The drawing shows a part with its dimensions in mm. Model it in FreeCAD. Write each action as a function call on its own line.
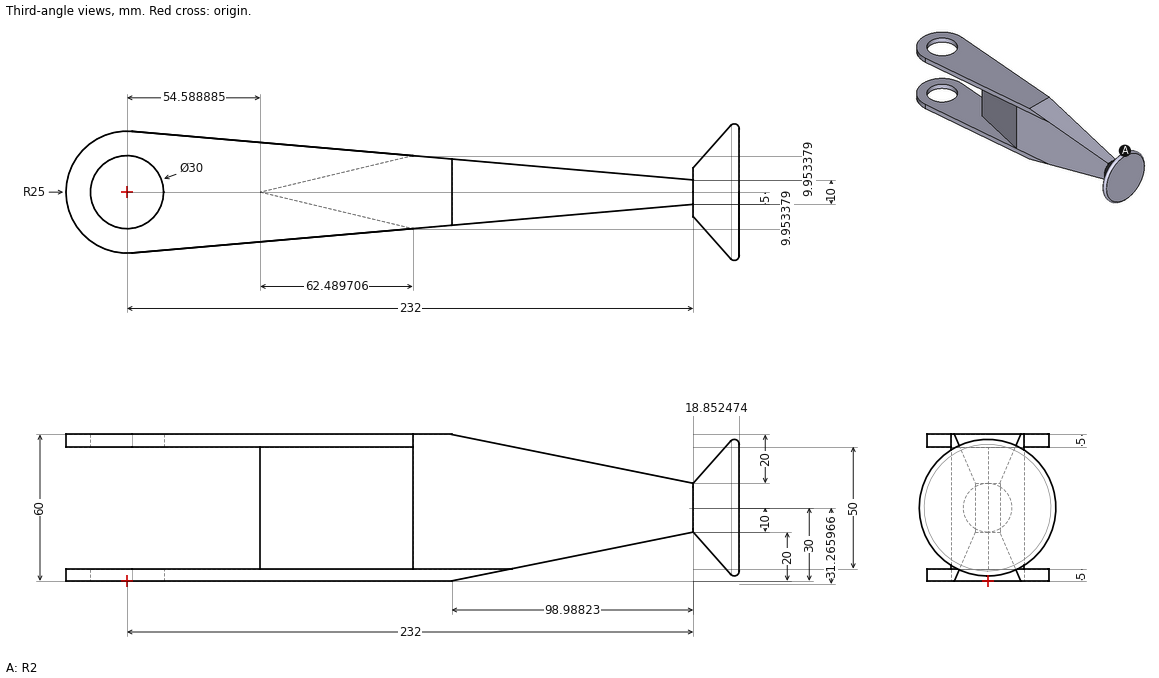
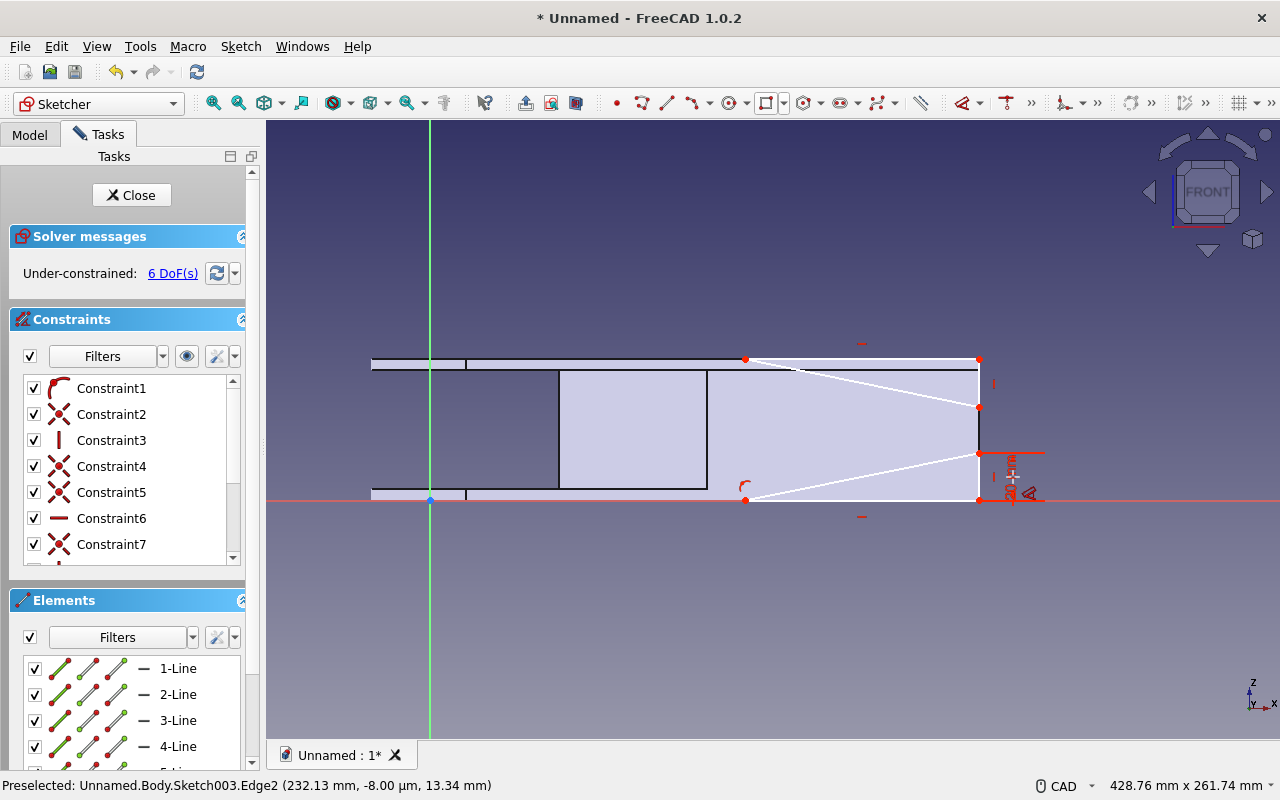
click(979, 374)
click(1013, 383)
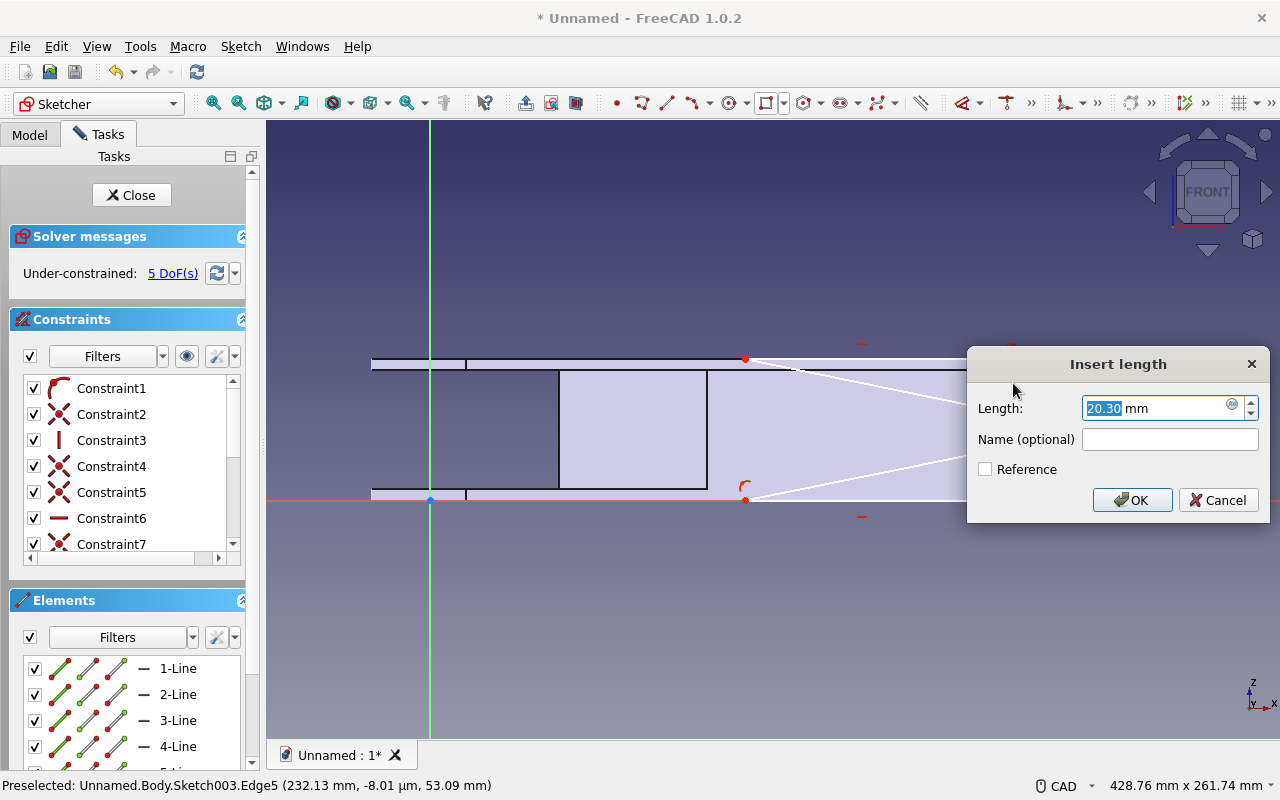
text(20)
key(Return)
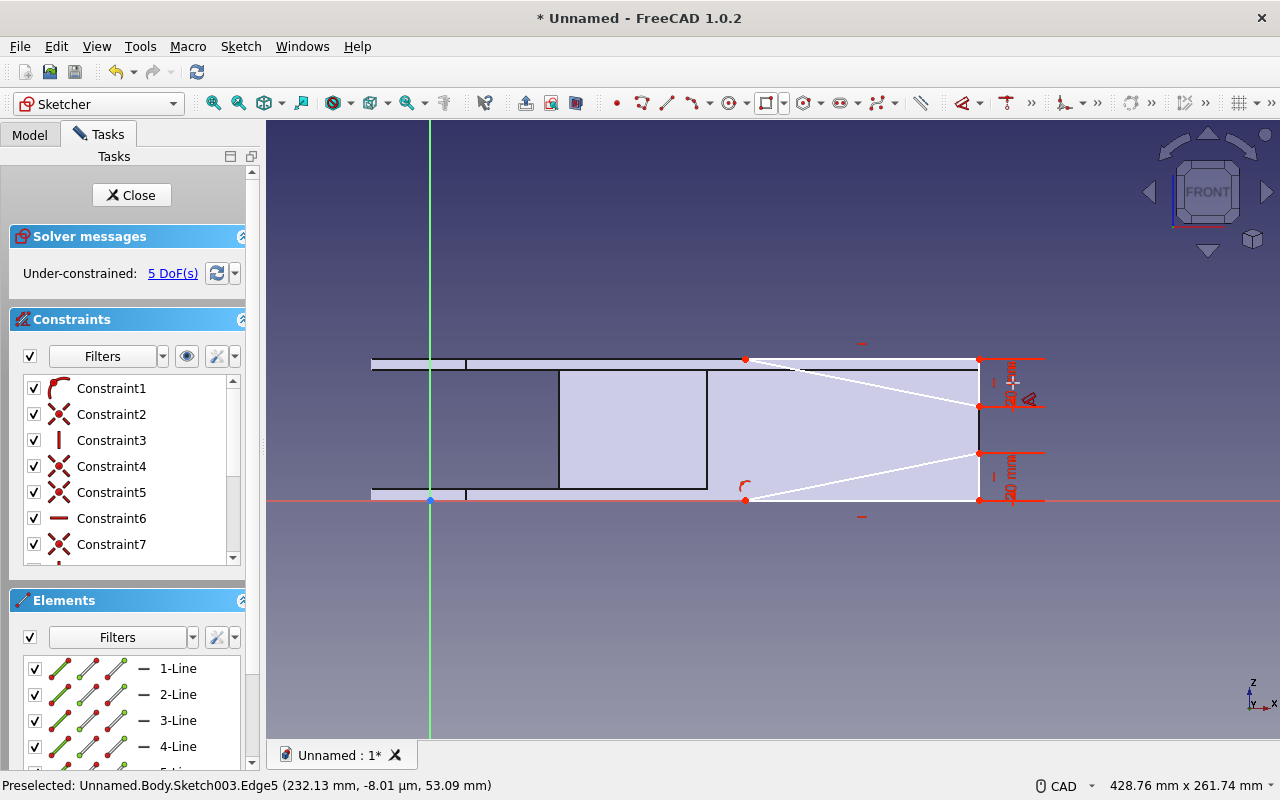
click(745, 359)
click(396, 430)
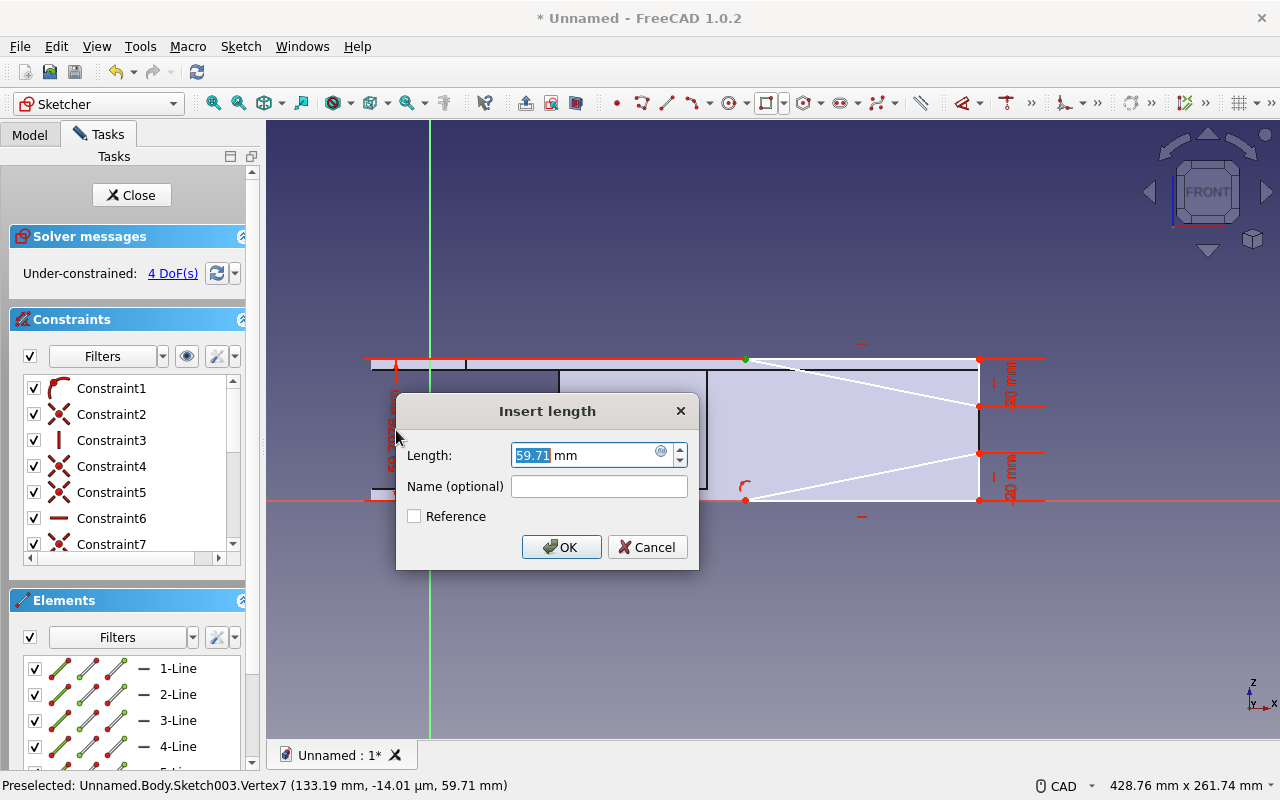
text(60)
key(Return)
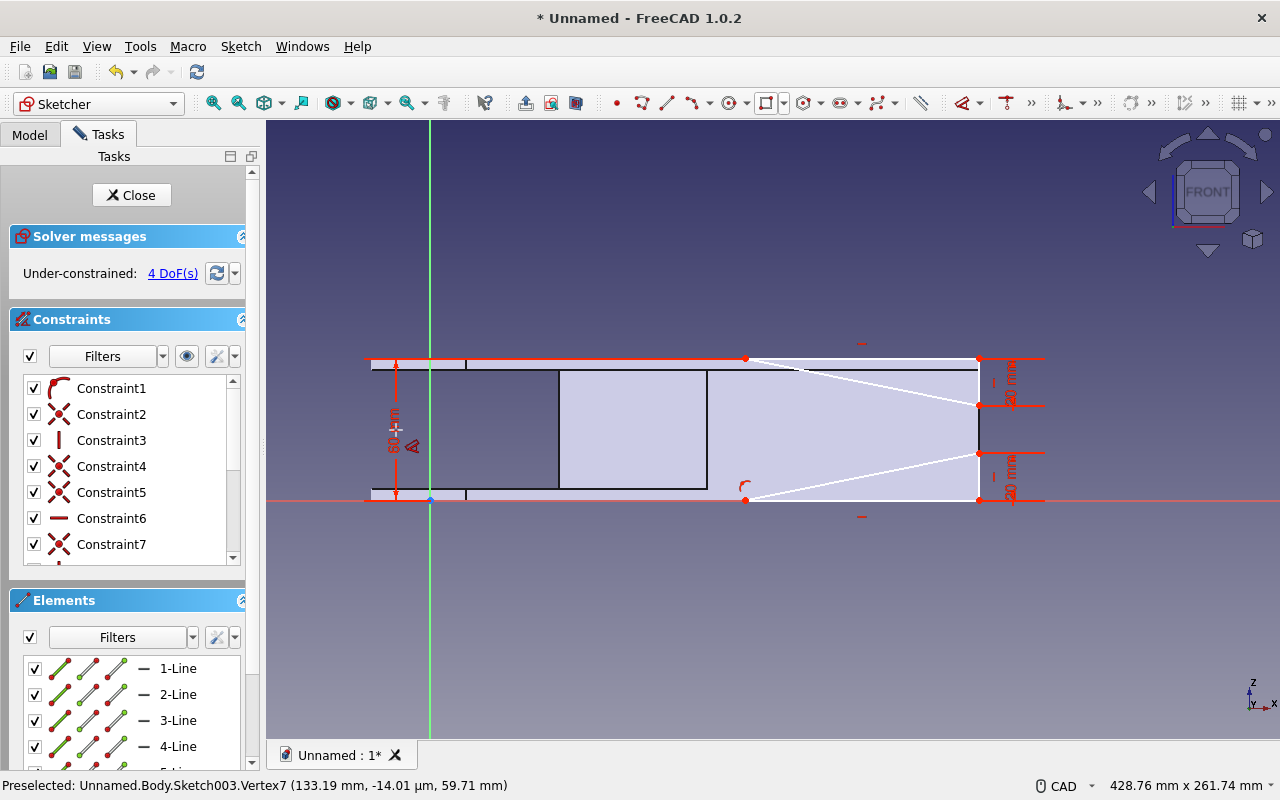
click(979, 453)
click(705, 535)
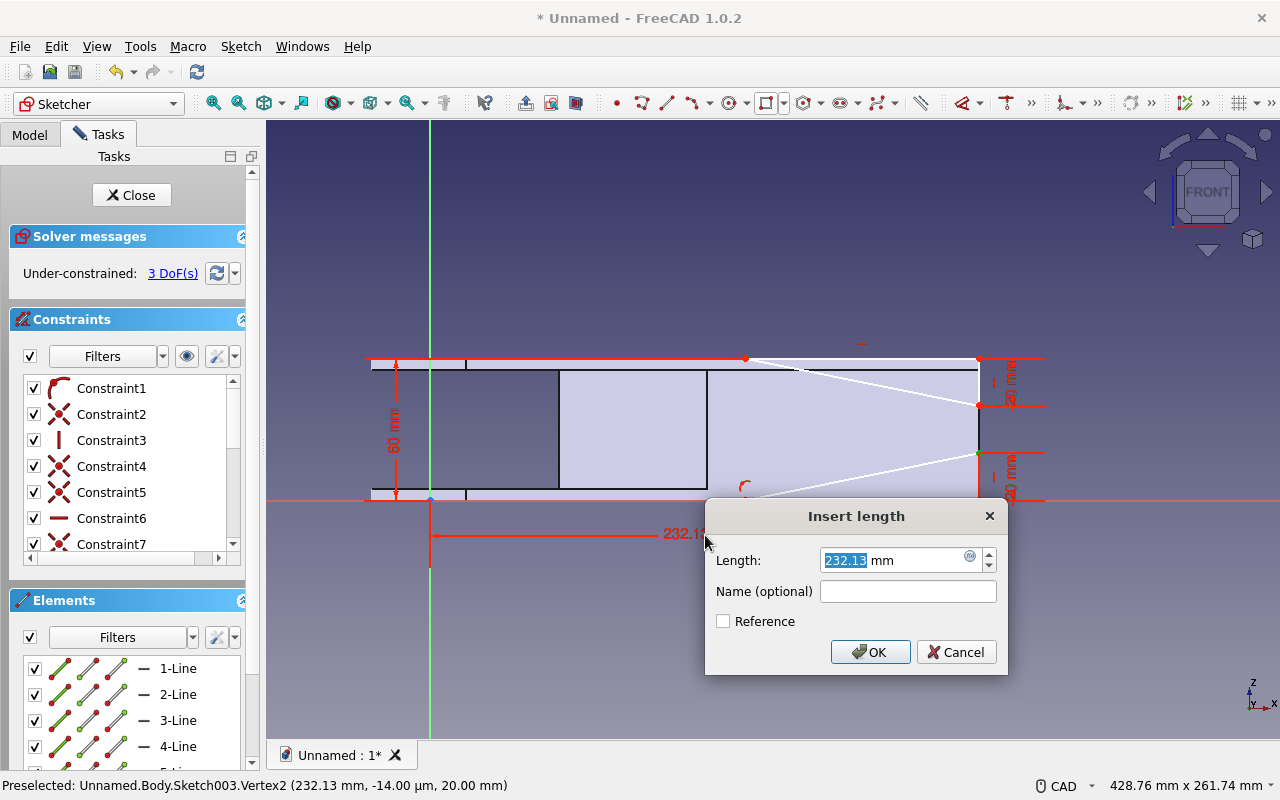
text(232)
key(Return)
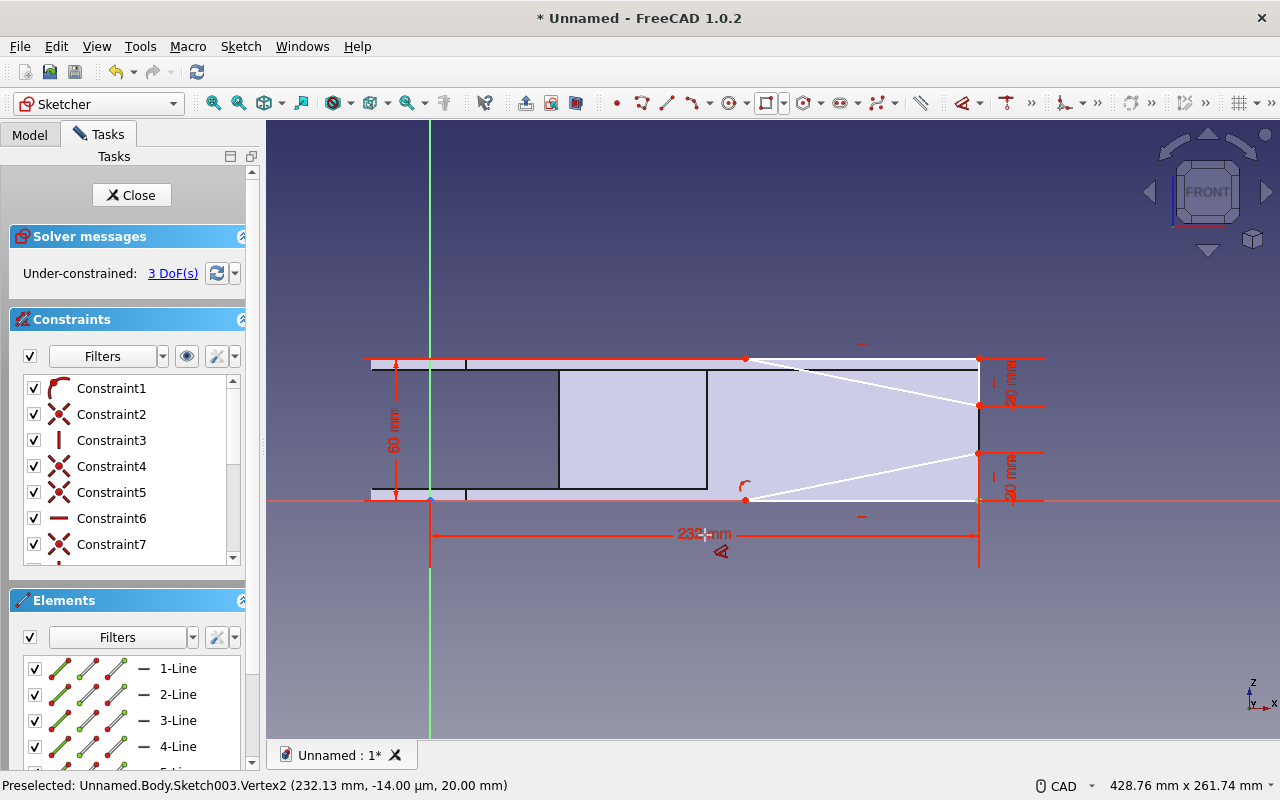
click(979, 359)
click(578, 535)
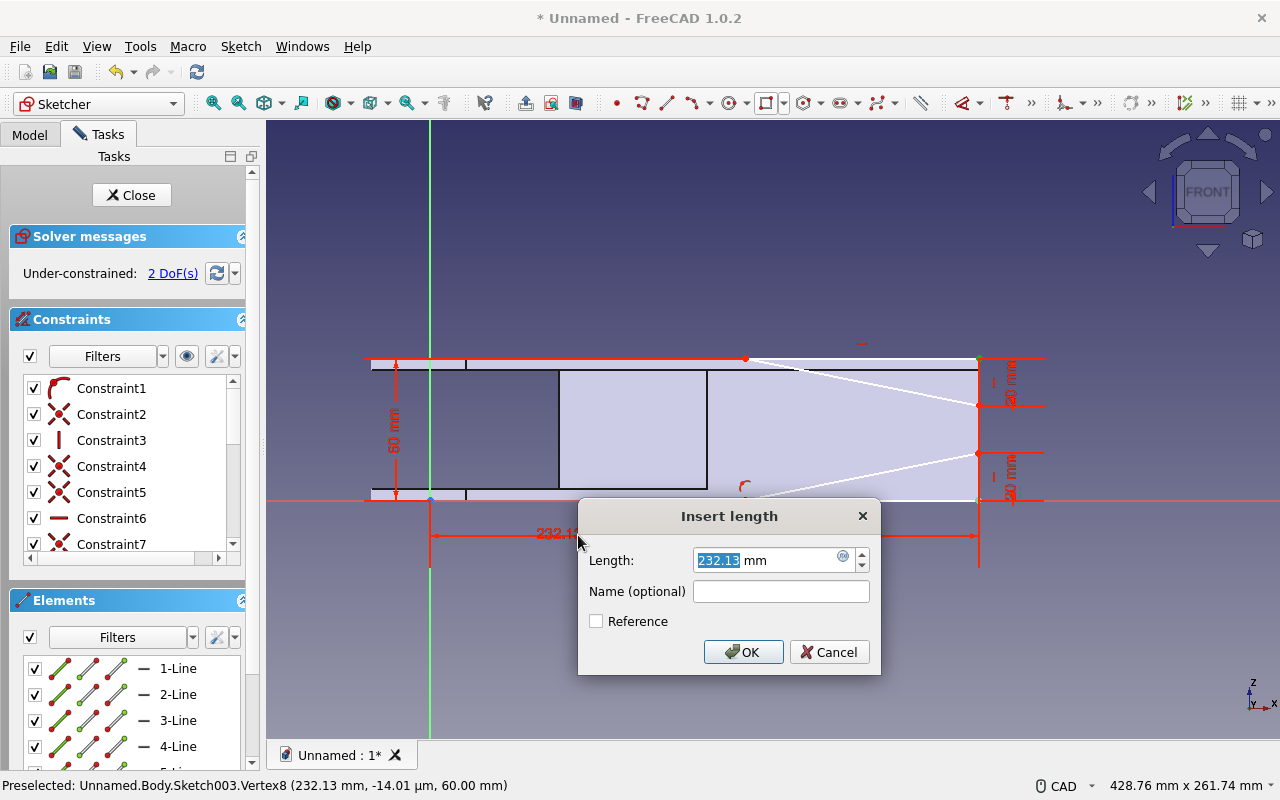
text(232)
key(Return)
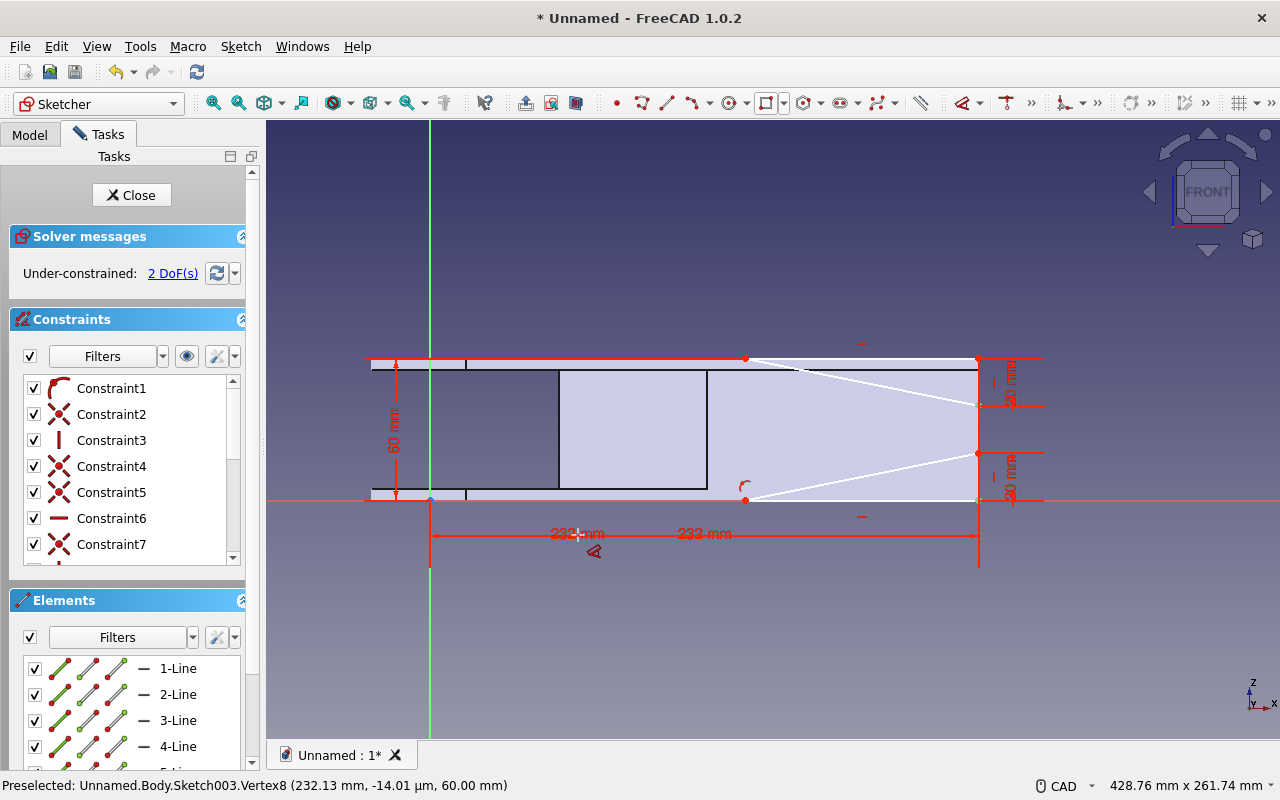
click(909, 501)
click(862, 535)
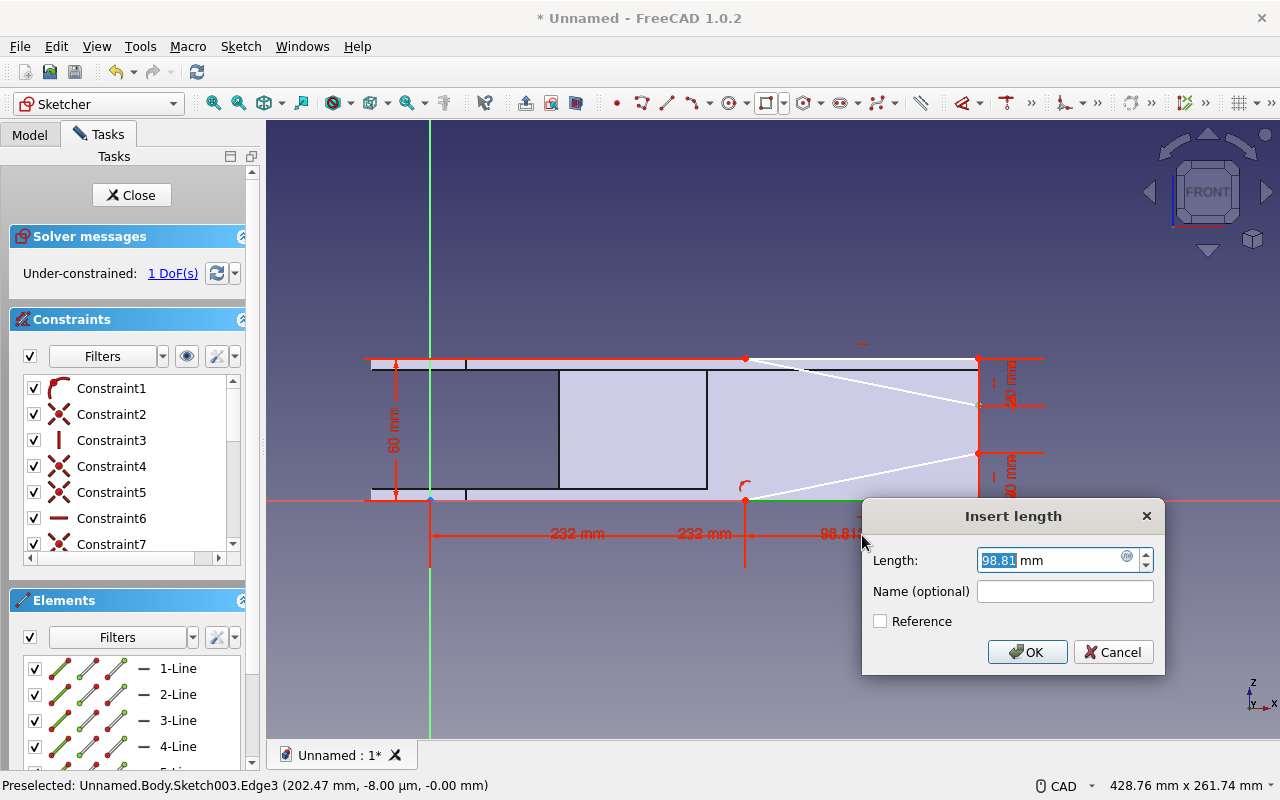
text(98.98823)
key(Return)